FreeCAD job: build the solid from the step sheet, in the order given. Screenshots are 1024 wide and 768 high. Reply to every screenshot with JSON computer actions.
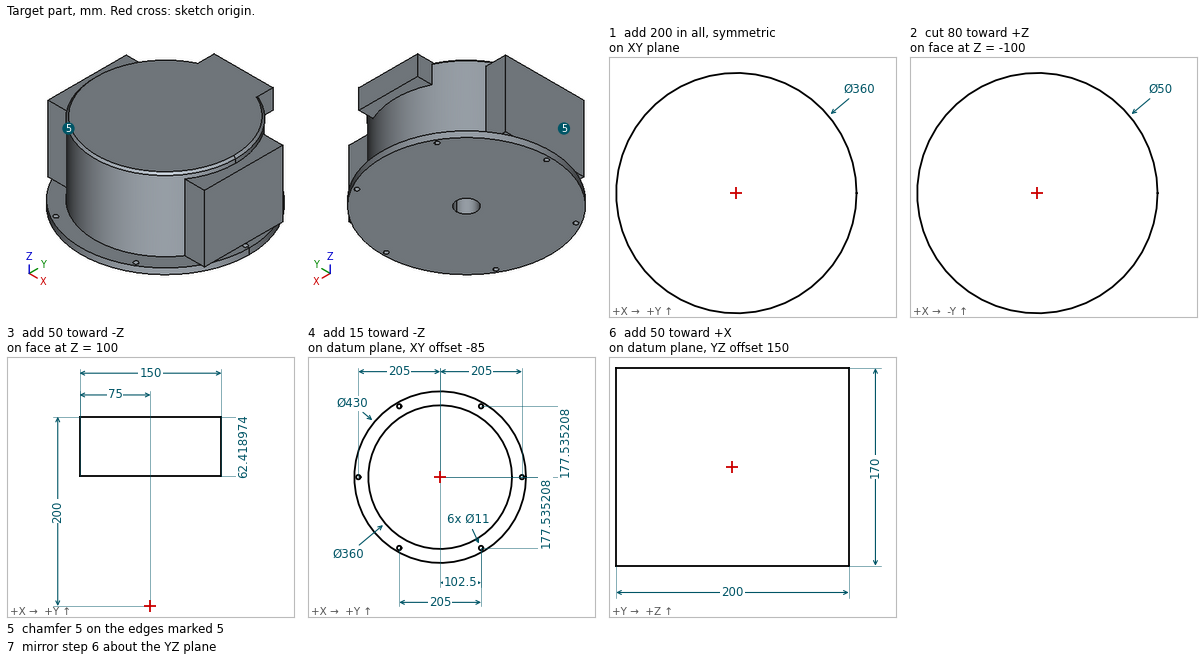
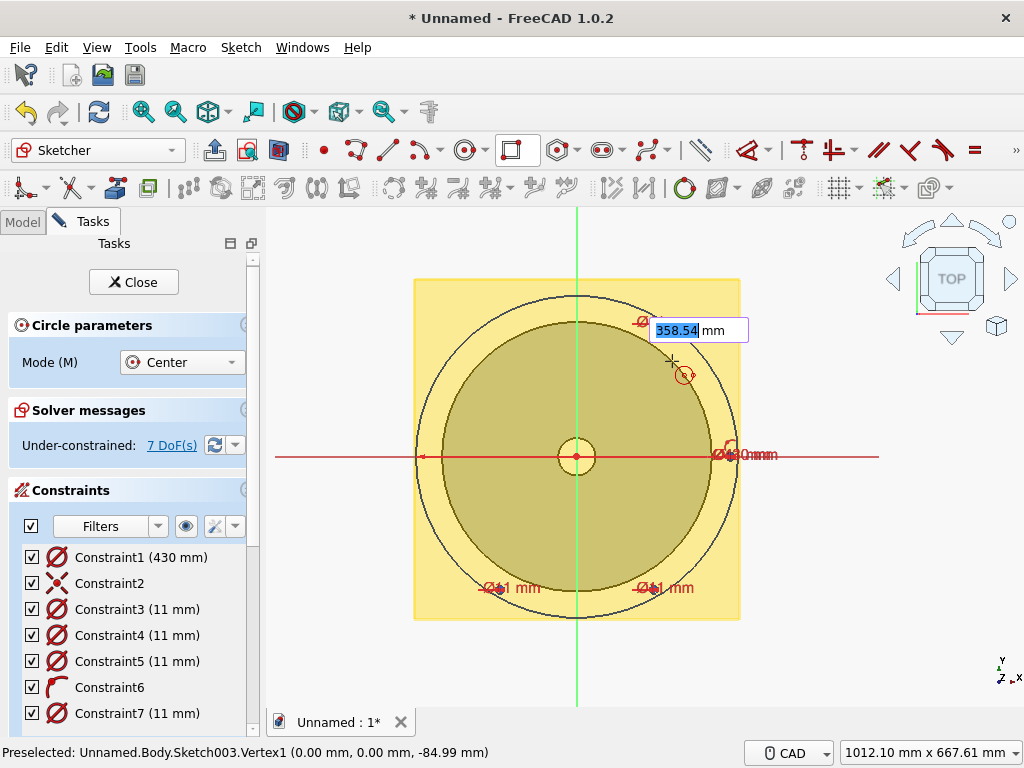
{"action": "type", "text": "360"}
{"action": "key", "text": "Return"}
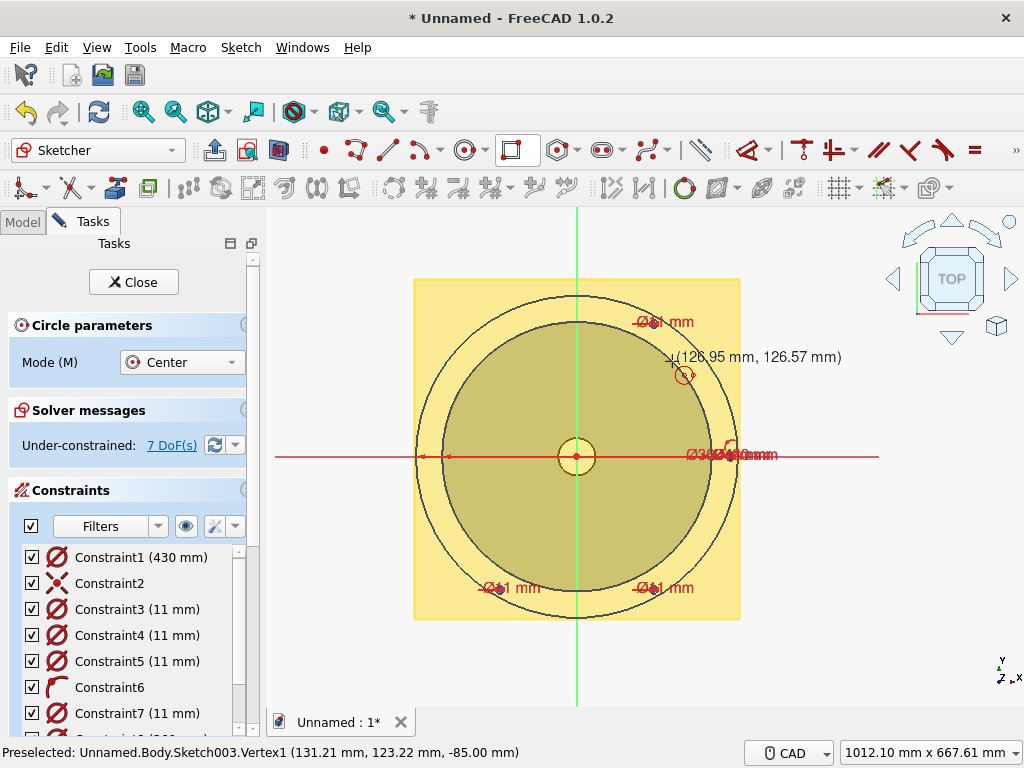
{"action": "scroll", "coordinate": [423, 457], "scroll_direction": "up", "scroll_amount": 9}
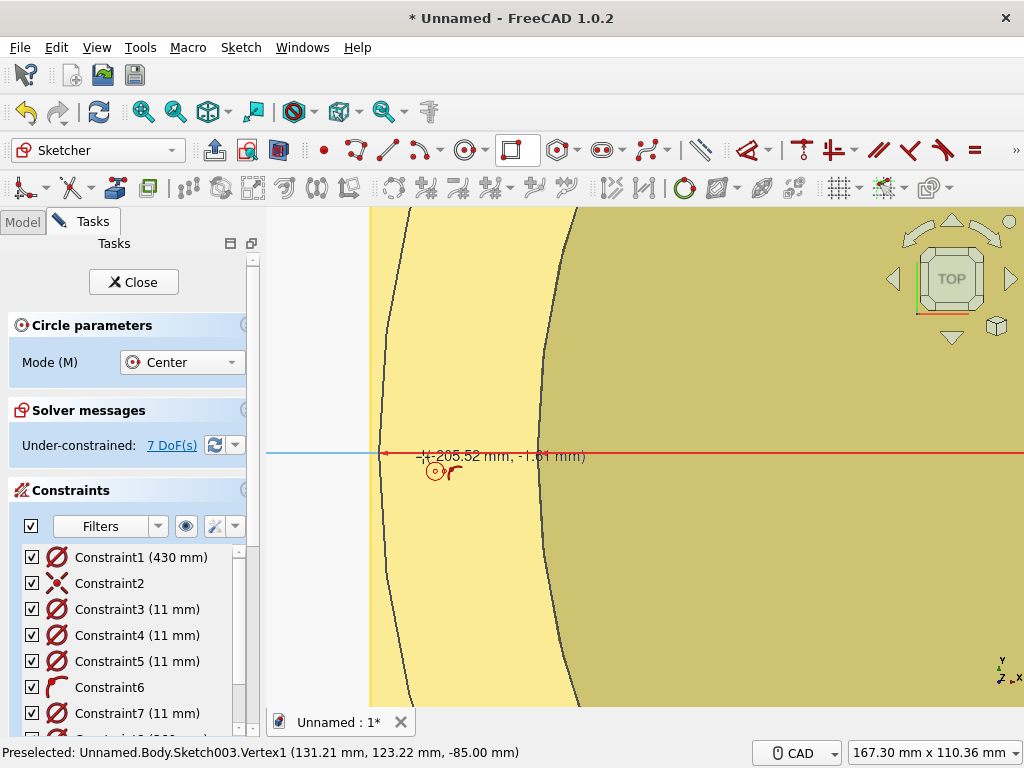
{"action": "left_click", "coordinate": [424, 453]}
{"action": "mouse_move", "coordinate": [442, 436]}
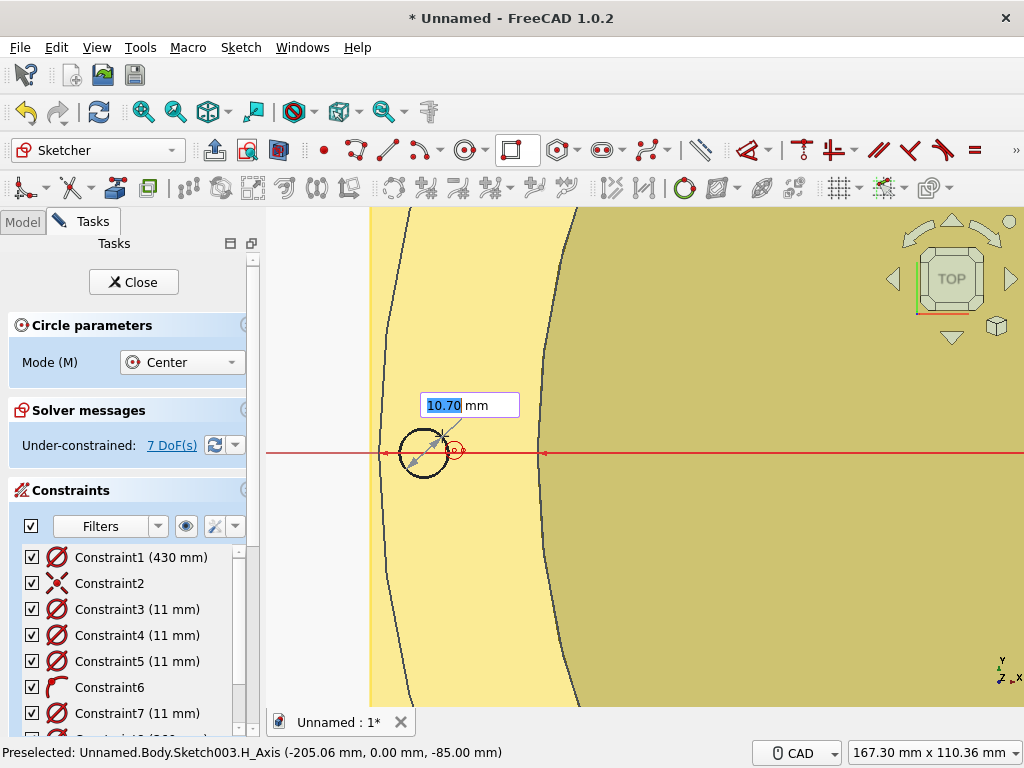
{"action": "type", "text": "11"}
{"action": "key", "text": "Return"}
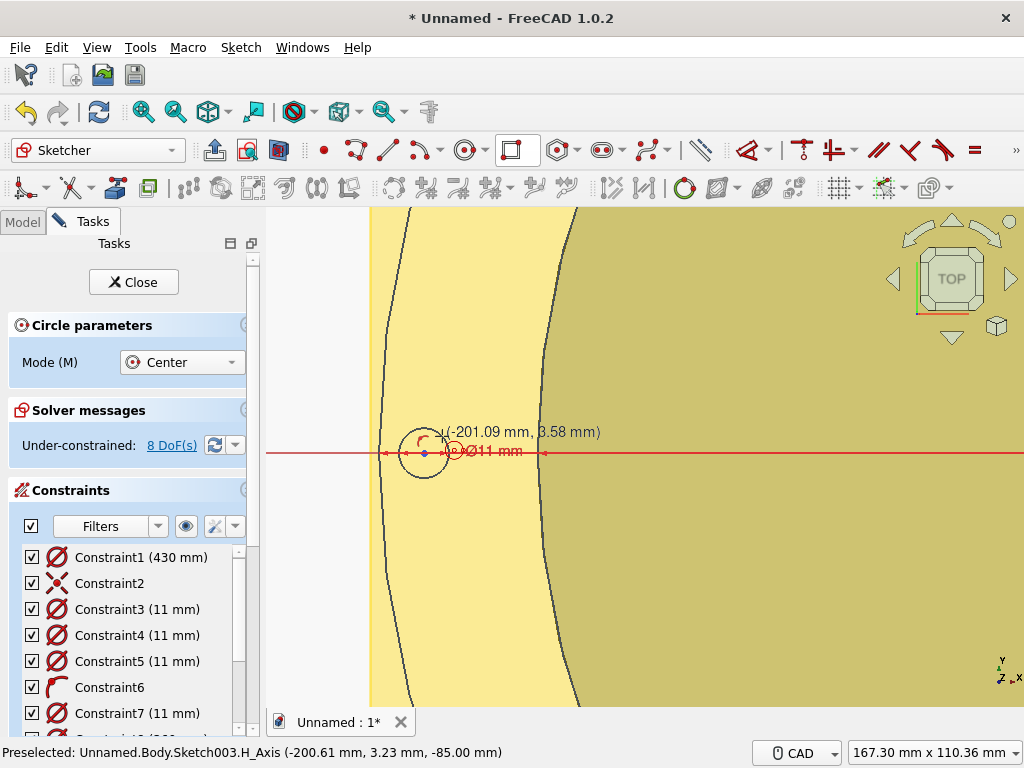
{"action": "scroll", "coordinate": [423, 458], "scroll_direction": "down", "scroll_amount": 9}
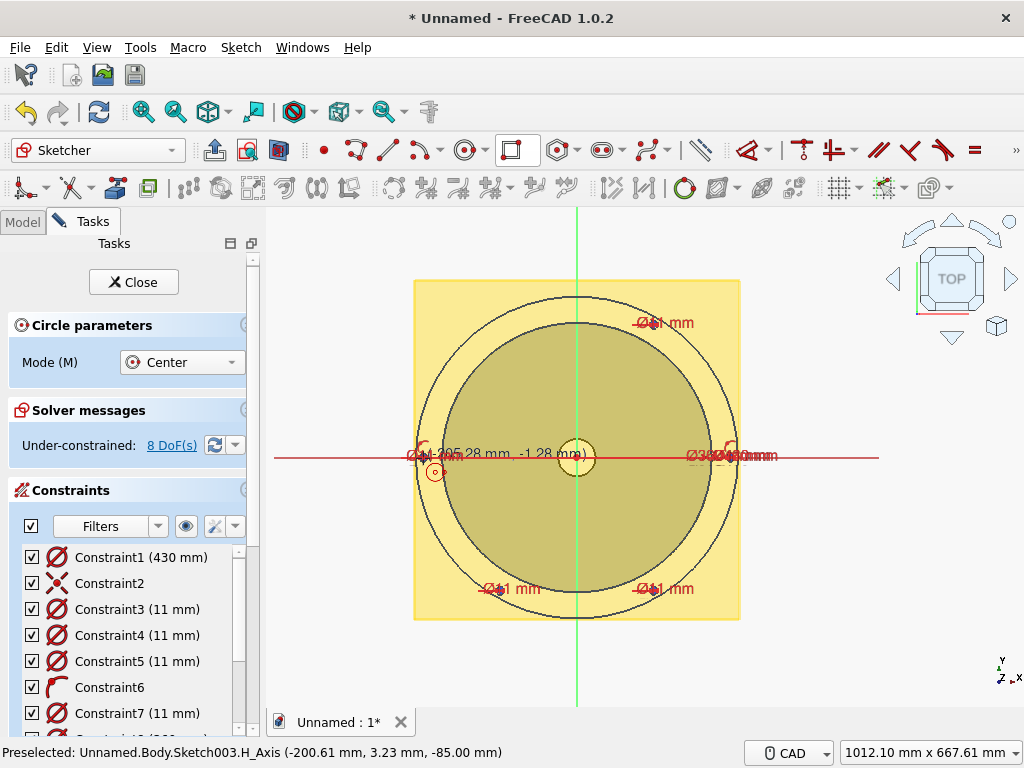
{"action": "scroll", "coordinate": [500, 325], "scroll_direction": "up", "scroll_amount": 9}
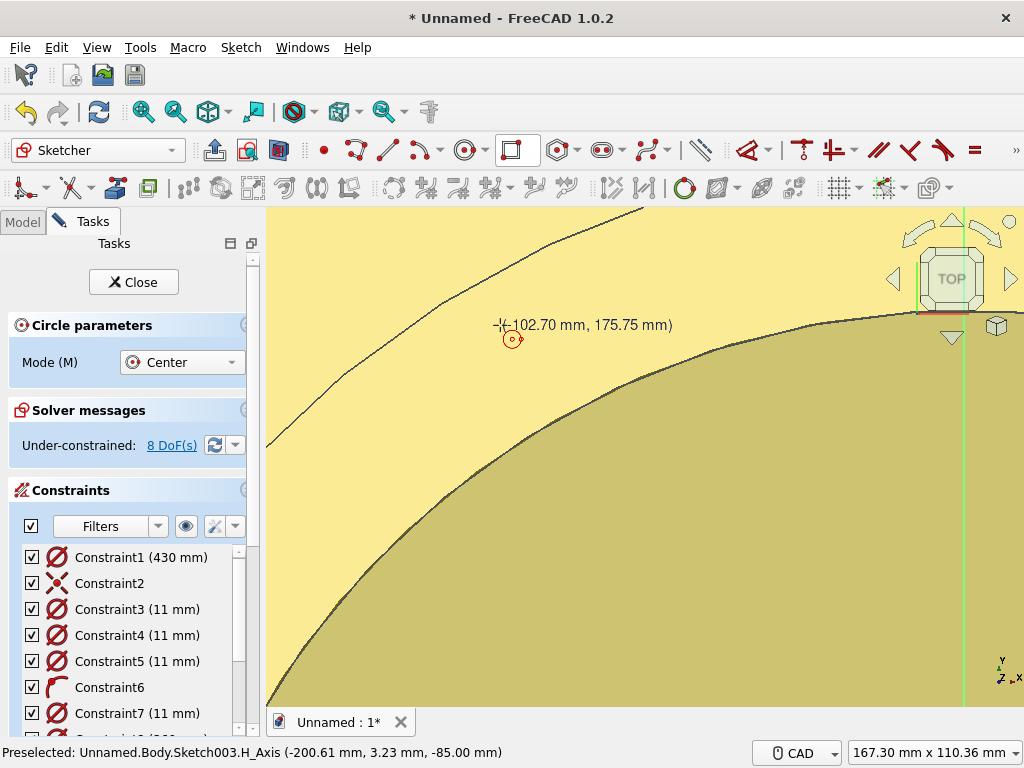
{"action": "left_click", "coordinate": [499, 322]}
{"action": "mouse_move", "coordinate": [517, 304]}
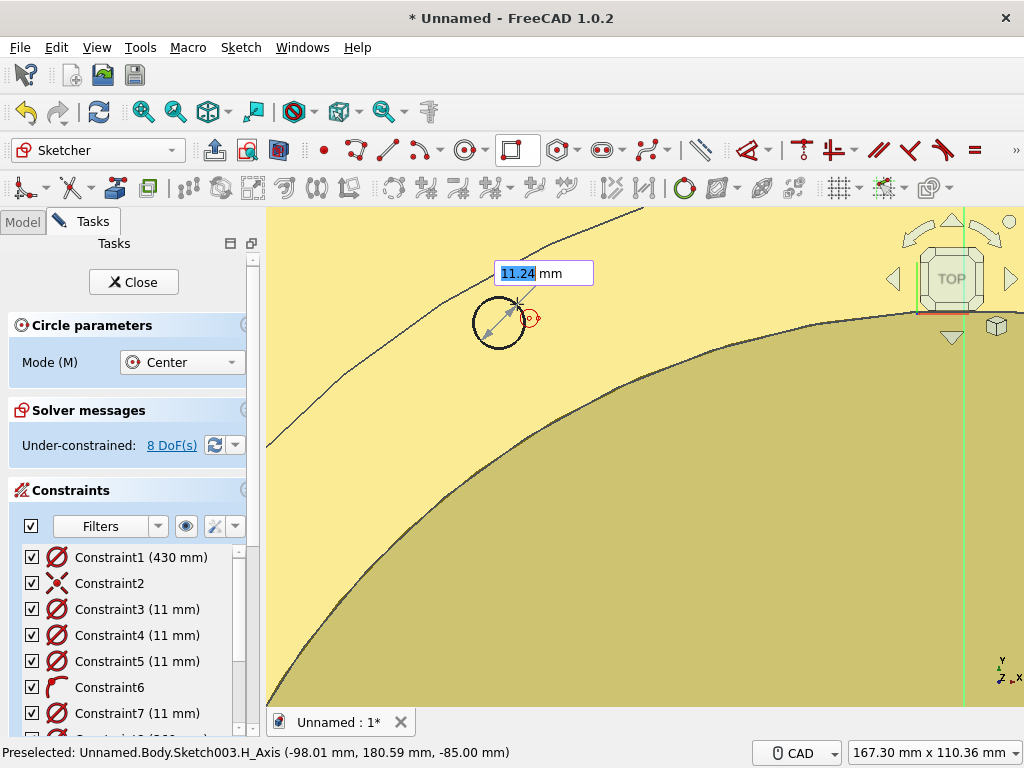
{"action": "type", "text": "11"}
{"action": "key", "text": "Return"}
{"action": "key", "text": "Escape"}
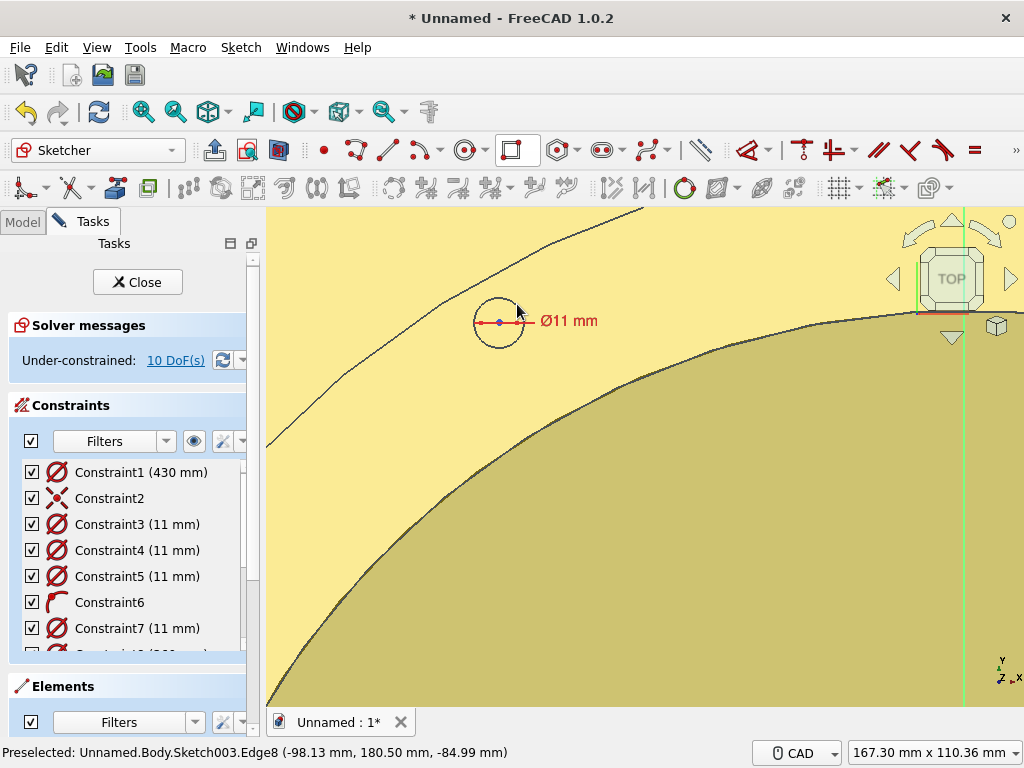
{"action": "scroll", "coordinate": [500, 324], "scroll_direction": "down", "scroll_amount": 9}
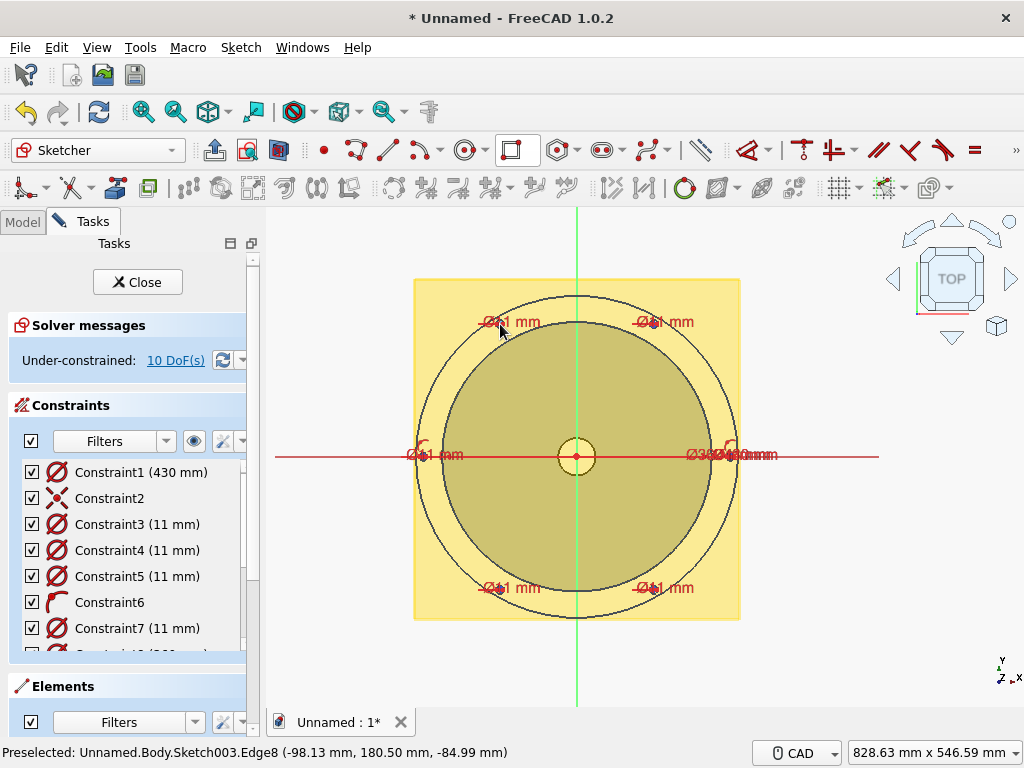
{"action": "left_click", "coordinate": [654, 590]}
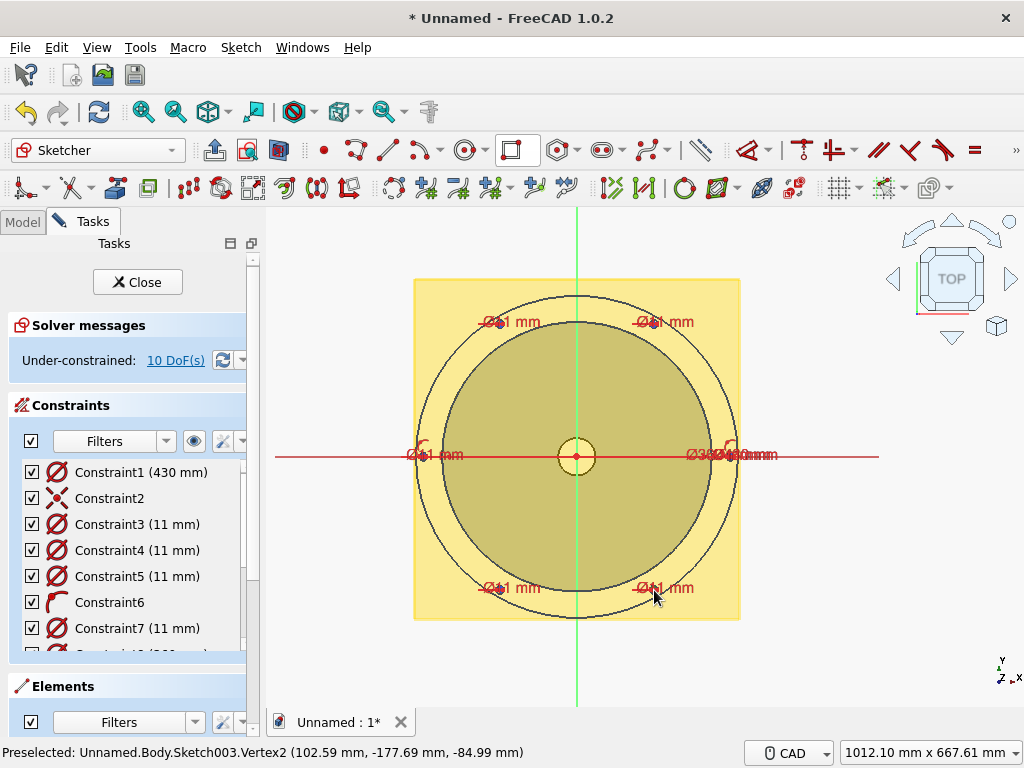
{"action": "left_click", "coordinate": [500, 590]}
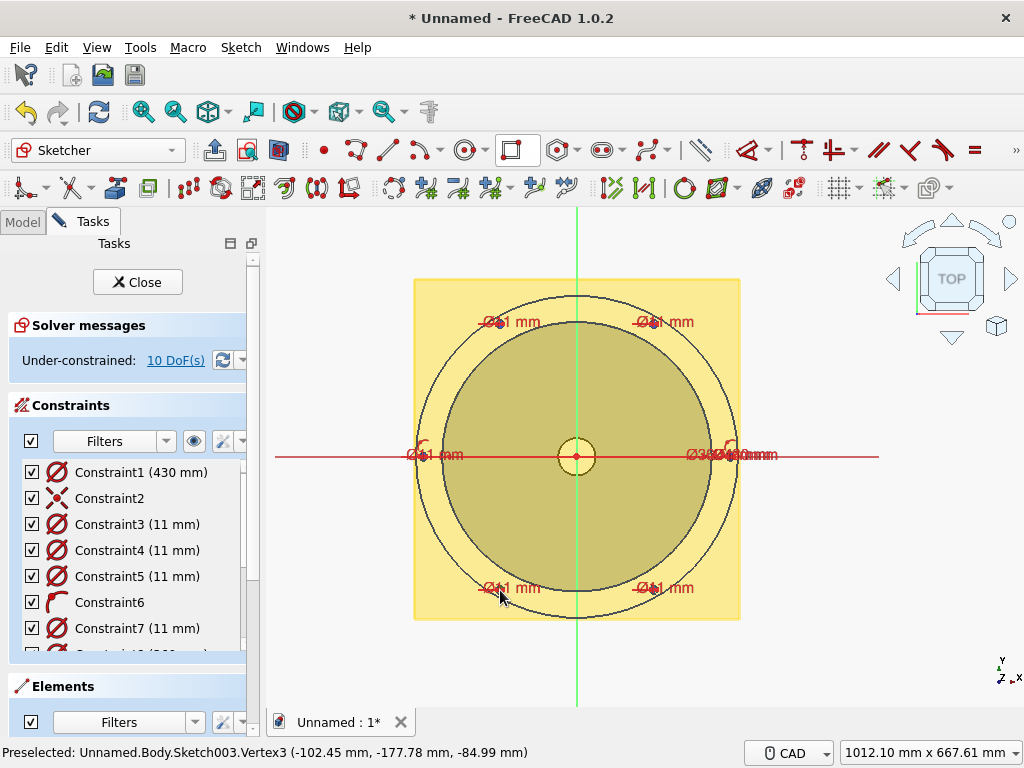
{"action": "key", "text": "h"}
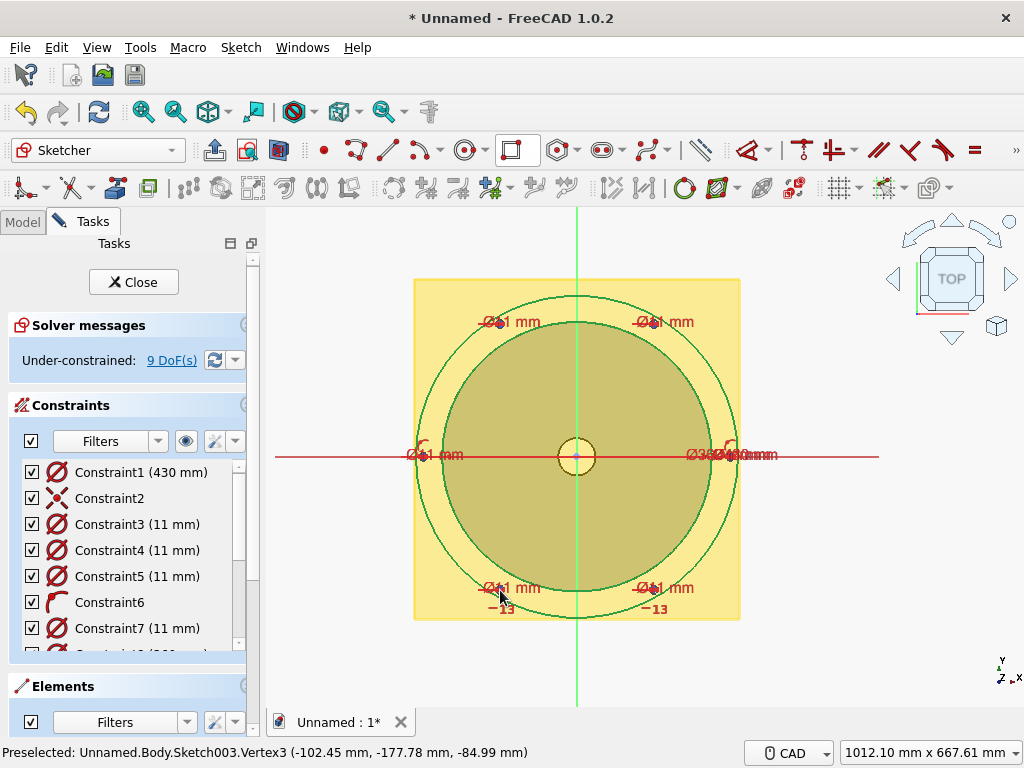
{"action": "left_click", "coordinate": [654, 590]}